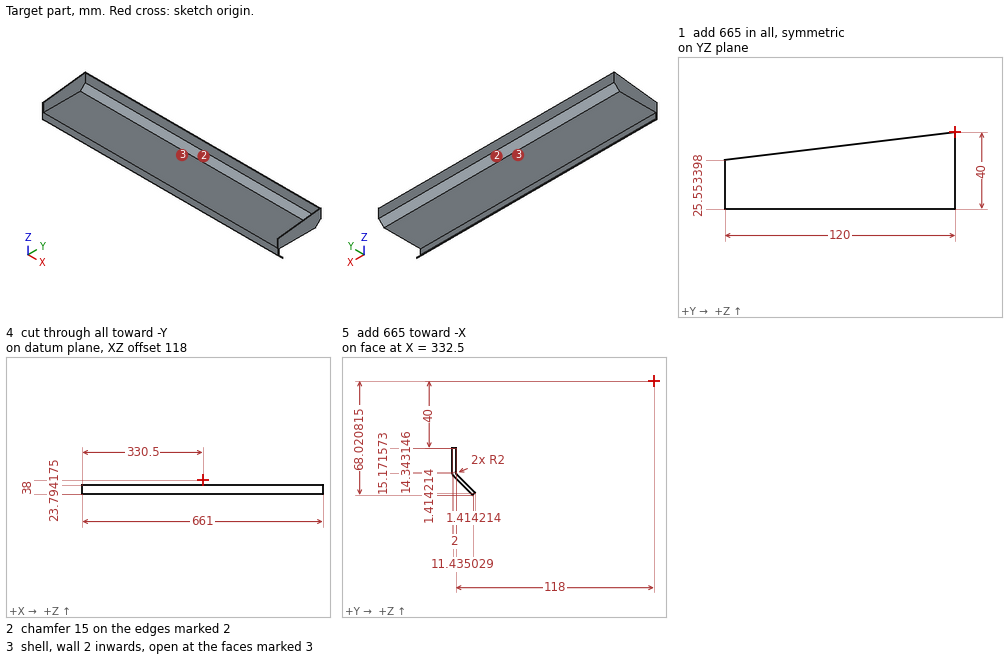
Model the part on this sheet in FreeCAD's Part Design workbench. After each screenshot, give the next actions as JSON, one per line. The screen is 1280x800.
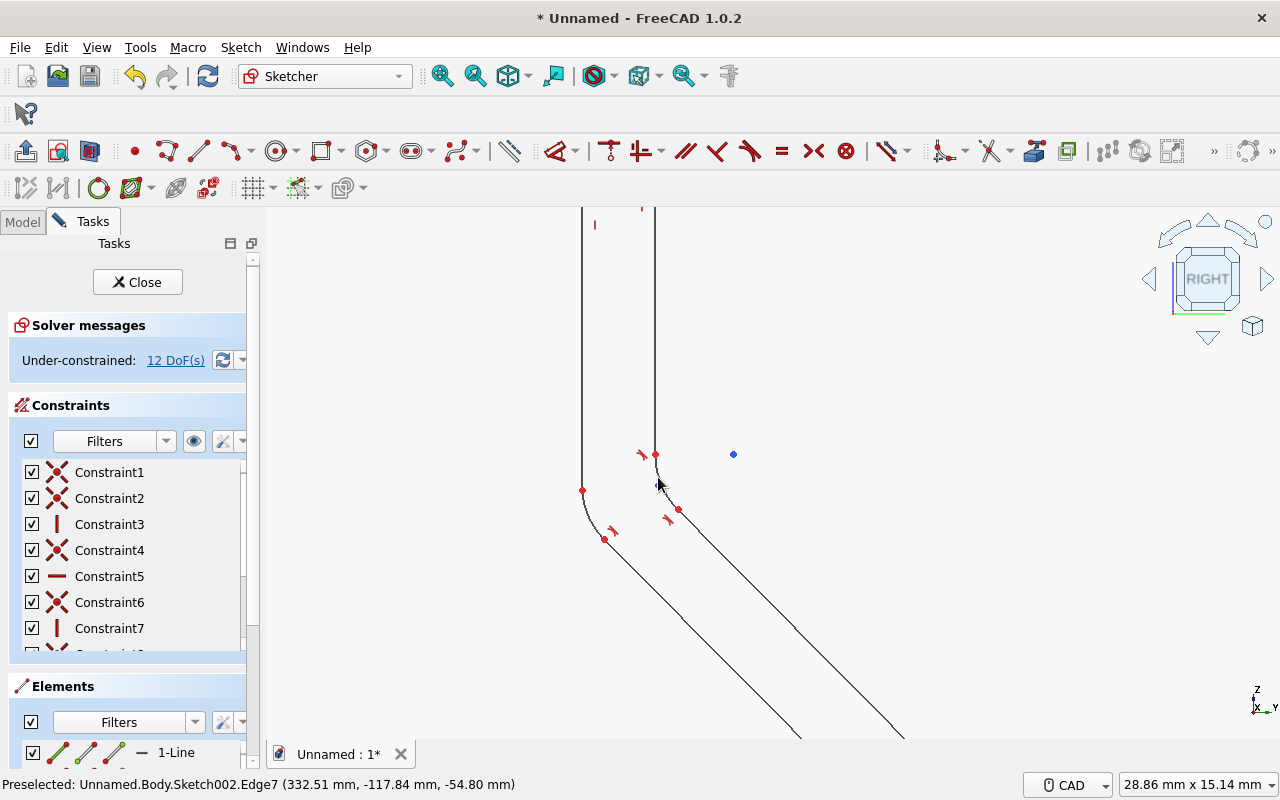
{"action": "left_click", "coordinate": [582, 331]}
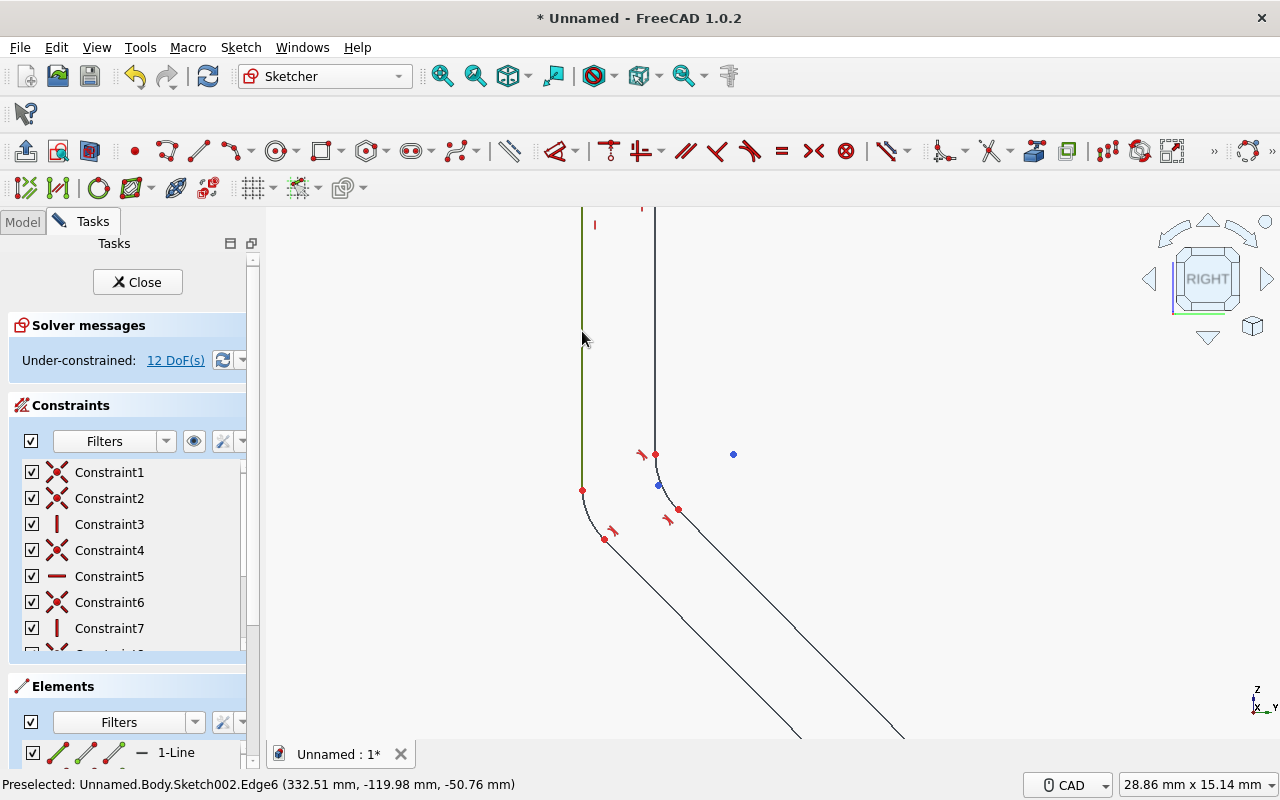
{"action": "left_click", "coordinate": [585, 507]}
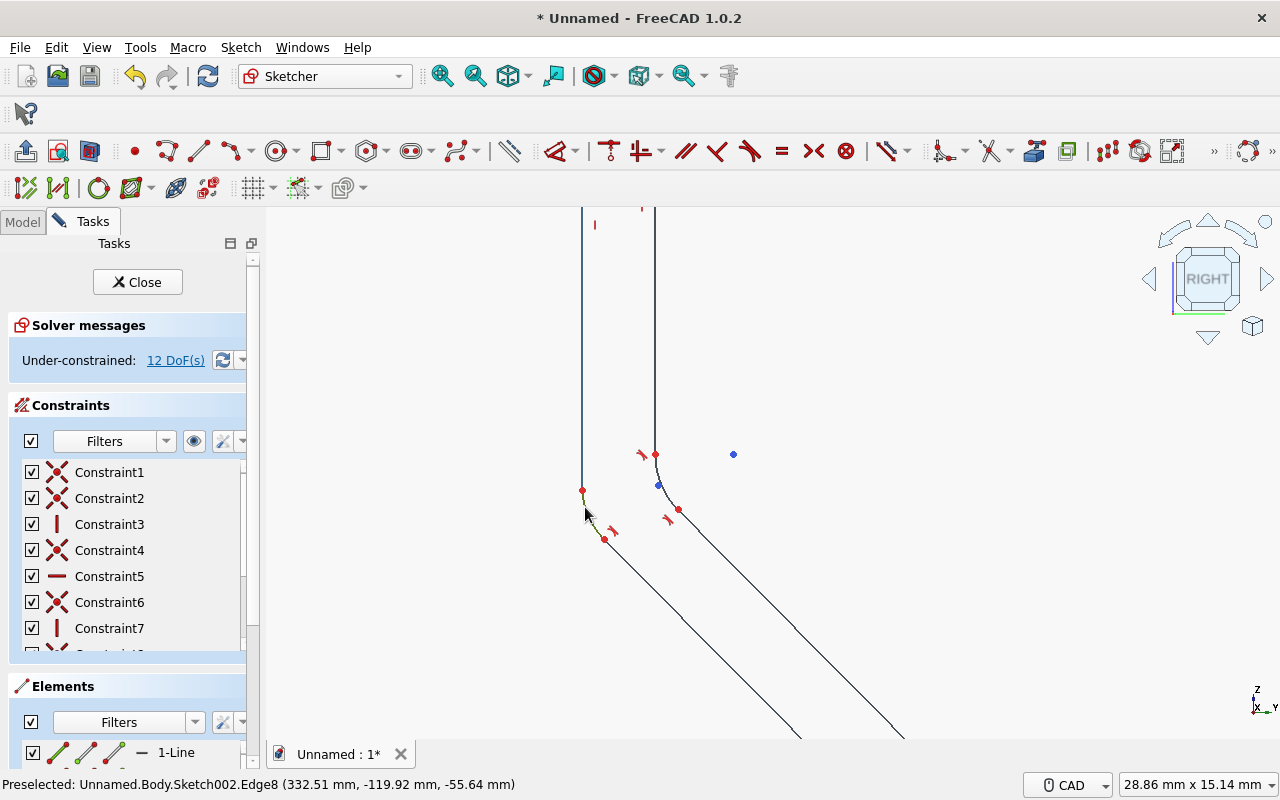
{"action": "key", "text": "t"}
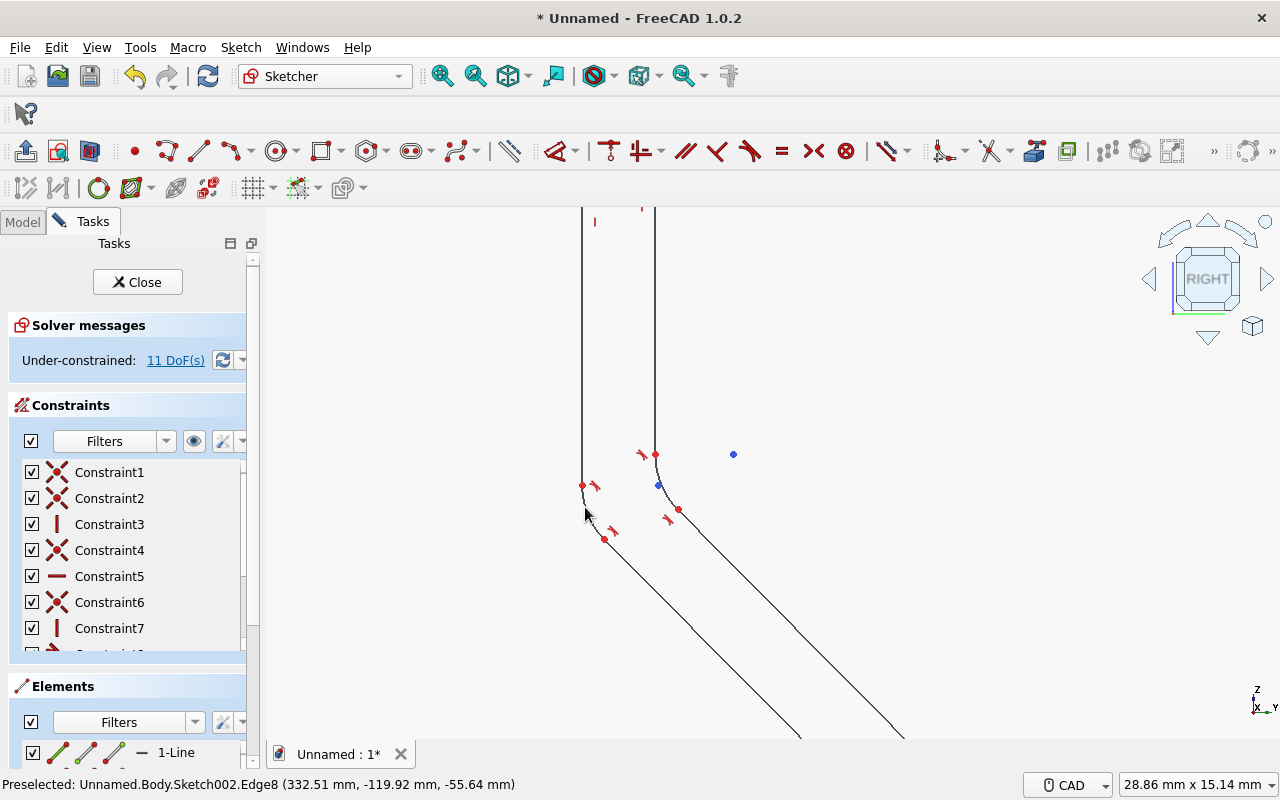
{"action": "left_click", "coordinate": [658, 473]}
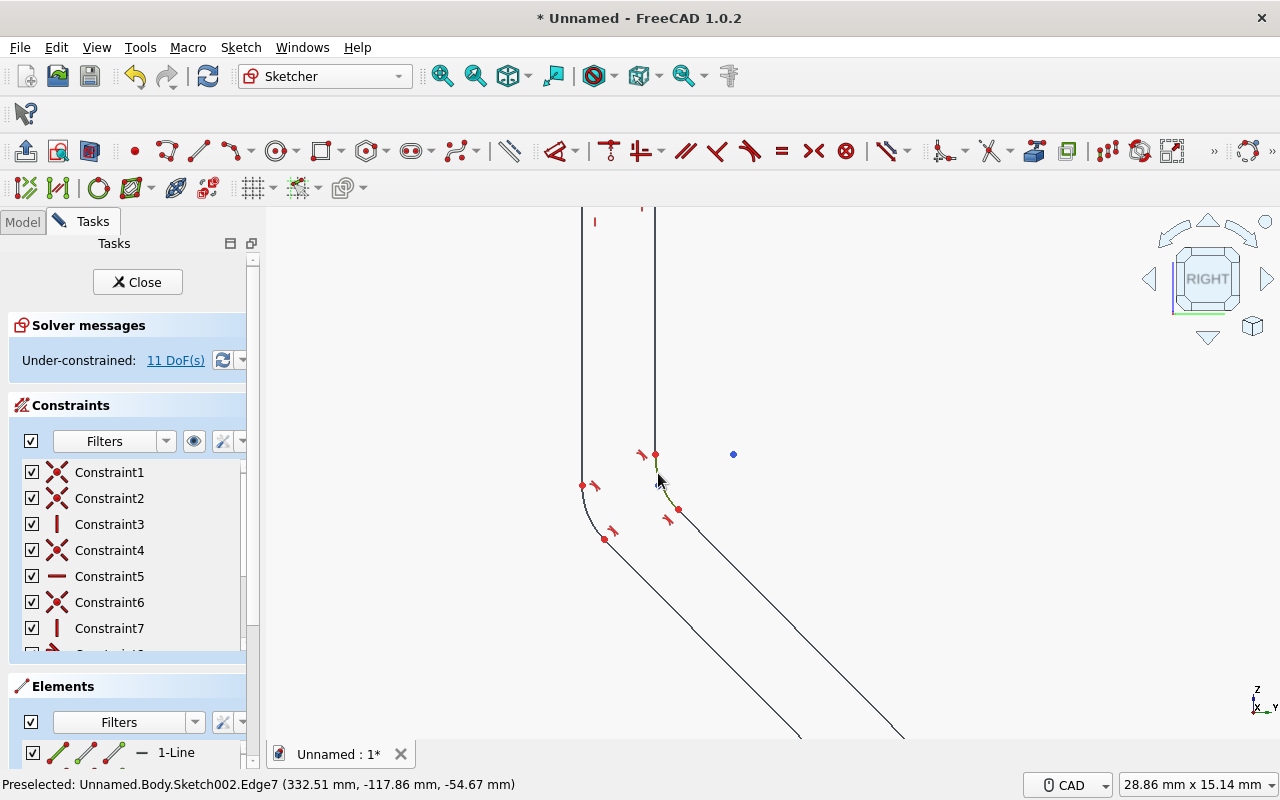
{"action": "left_click", "coordinate": [584, 504]}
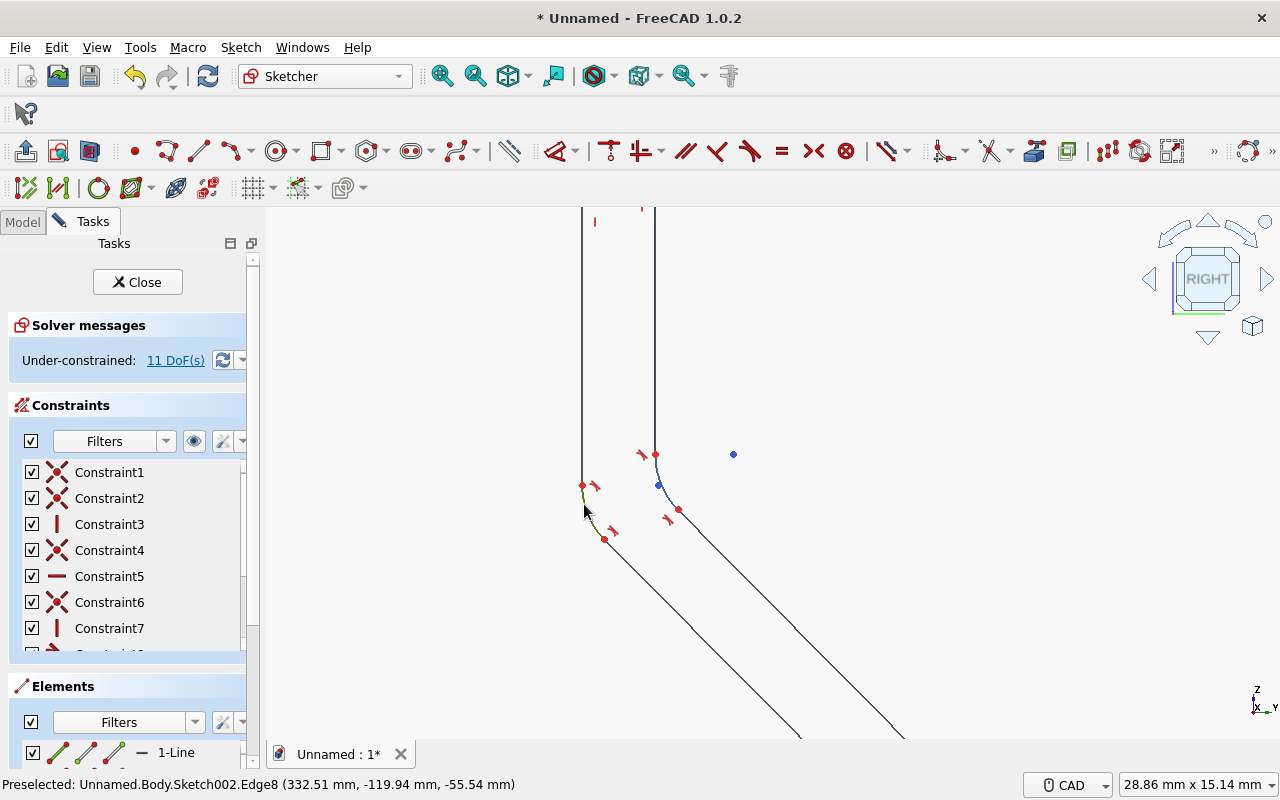
{"action": "left_click", "coordinate": [782, 152]}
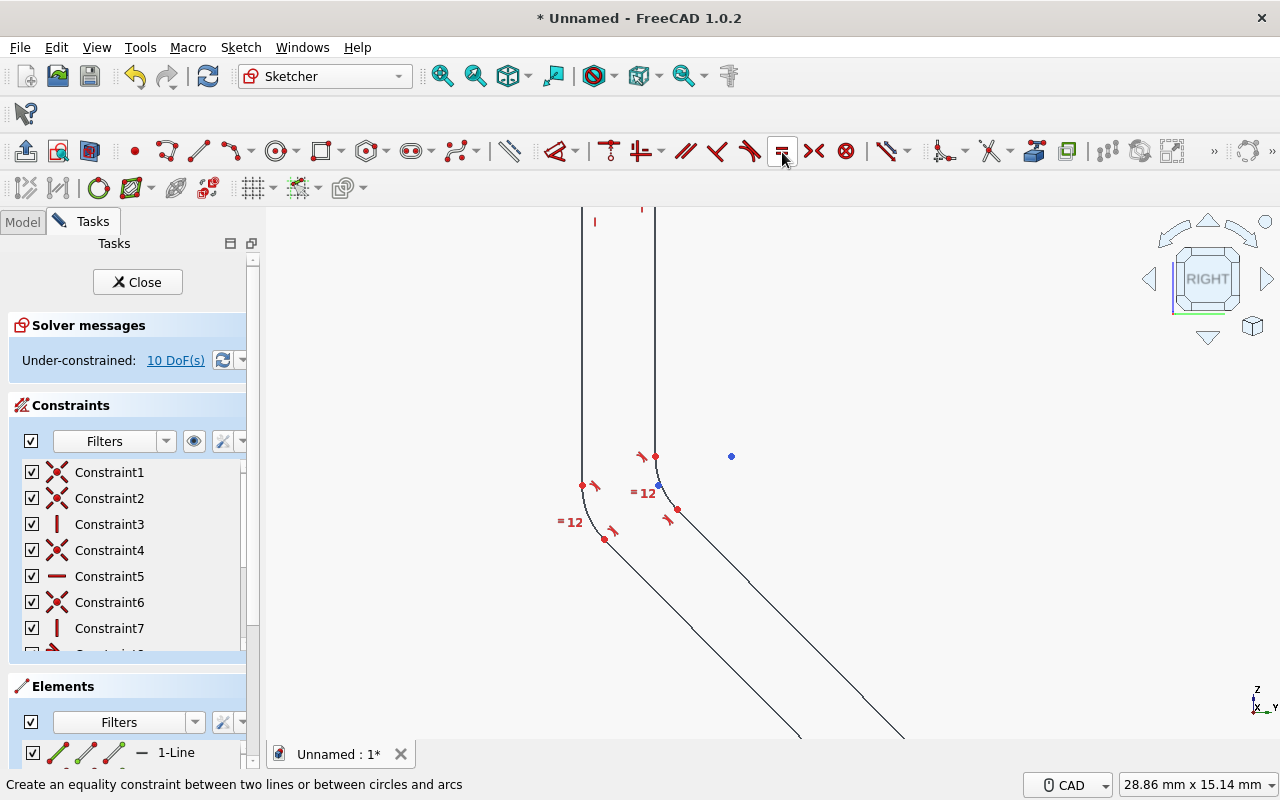
{"action": "key", "text": "d"}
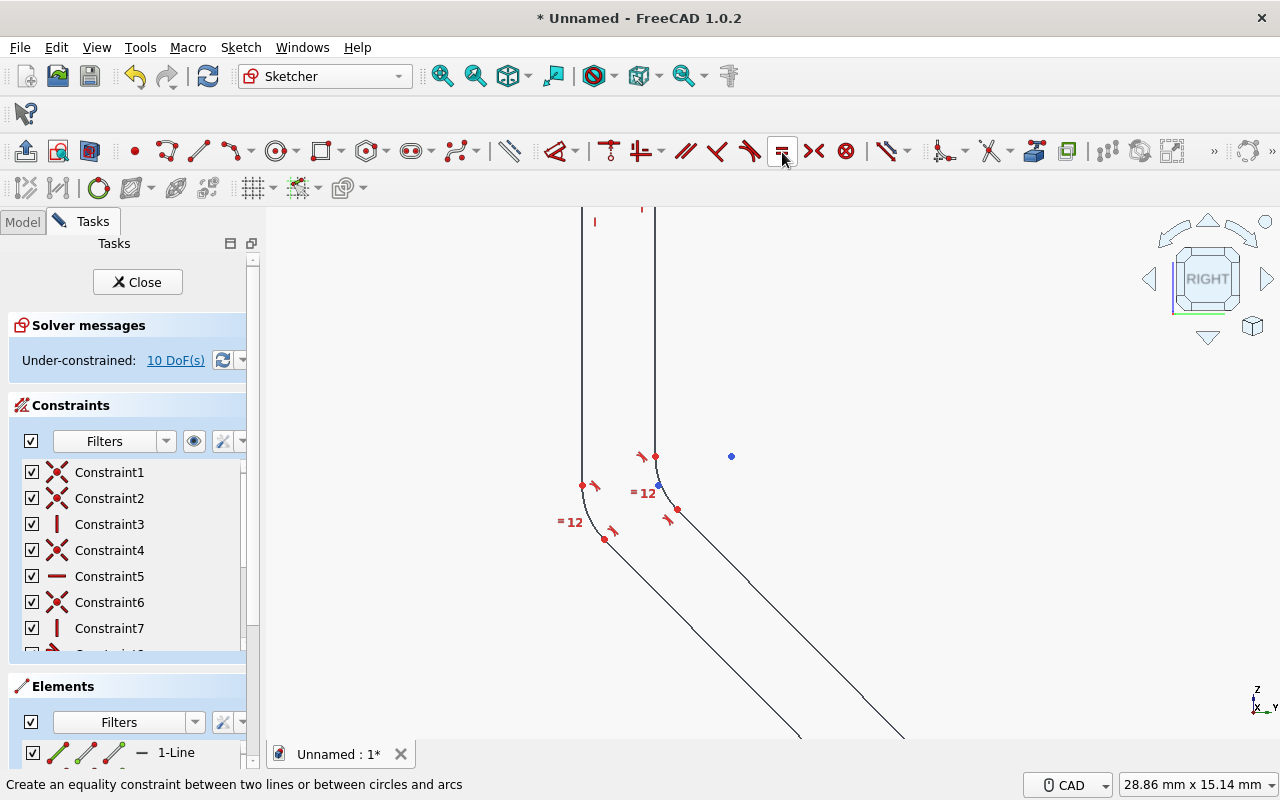
{"action": "left_click", "coordinate": [658, 474]}
{"action": "left_click", "coordinate": [627, 482]}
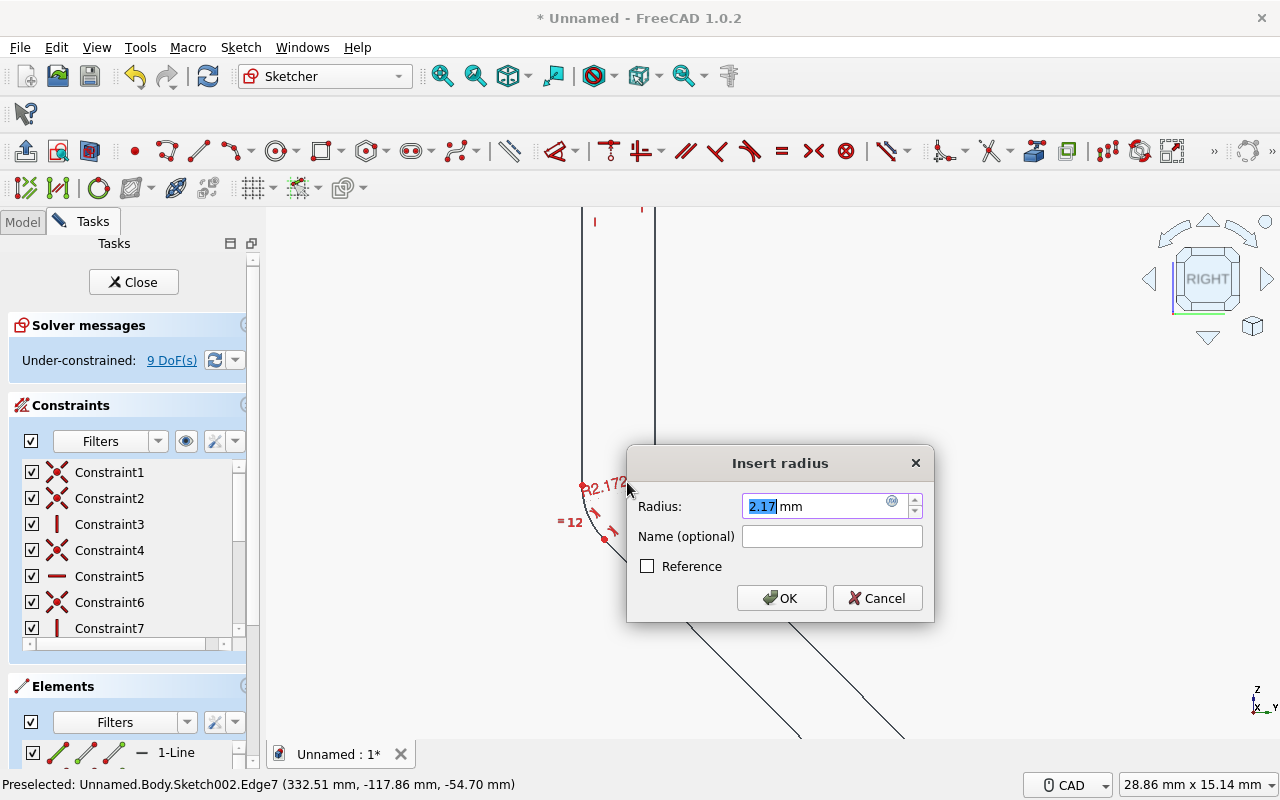
{"action": "type", "text": "2"}
{"action": "key", "text": "Return"}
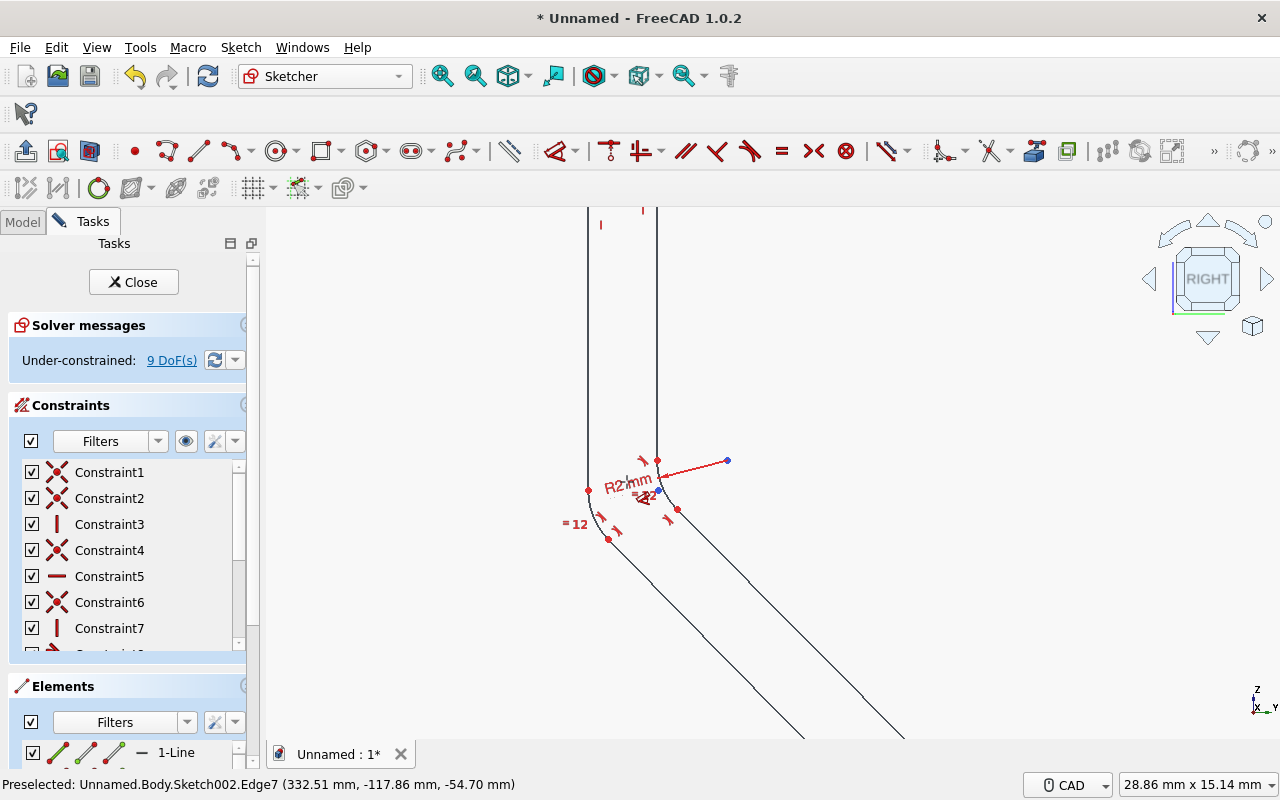
{"action": "scroll", "coordinate": [639, 489], "scroll_direction": "down", "scroll_amount": 5}